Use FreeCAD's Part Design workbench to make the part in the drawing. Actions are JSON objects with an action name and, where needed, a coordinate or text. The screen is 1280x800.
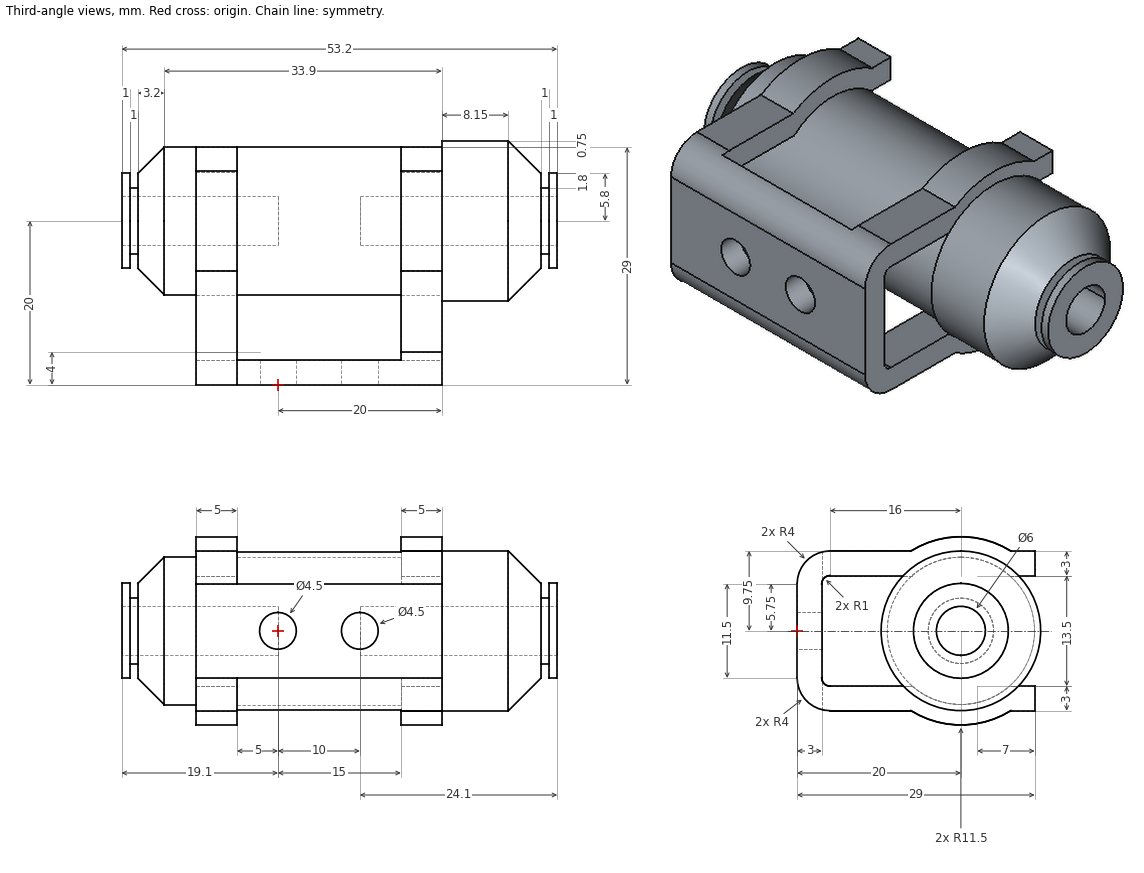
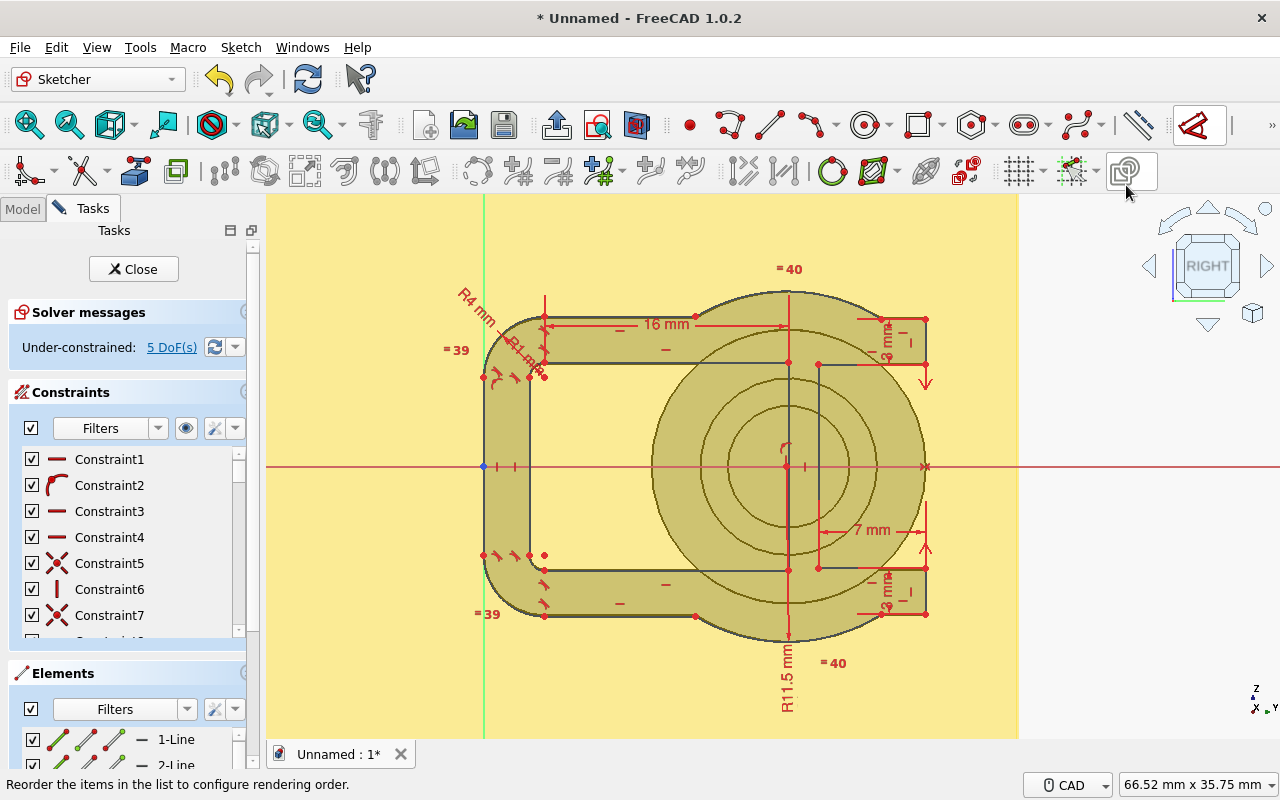
{"action": "left_click", "coordinate": [926, 614]}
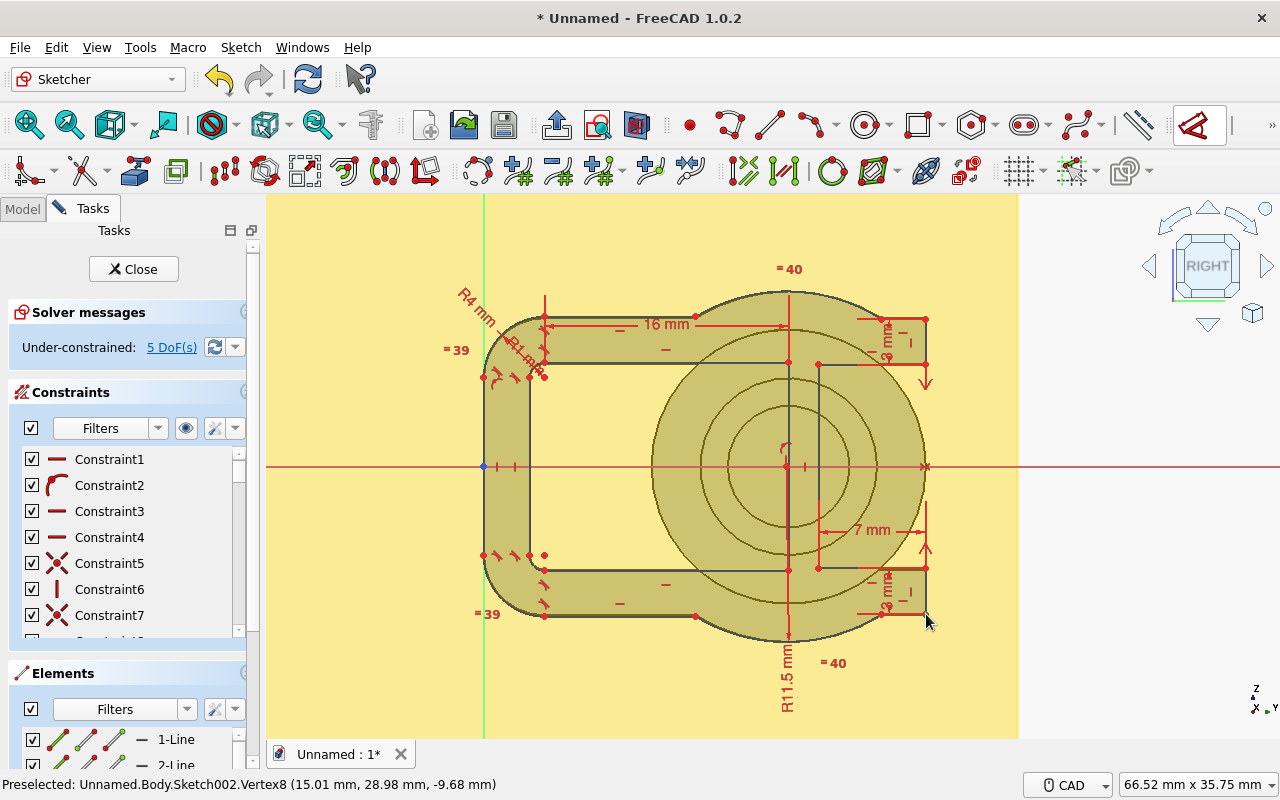
{"action": "left_click", "coordinate": [1220, 126]}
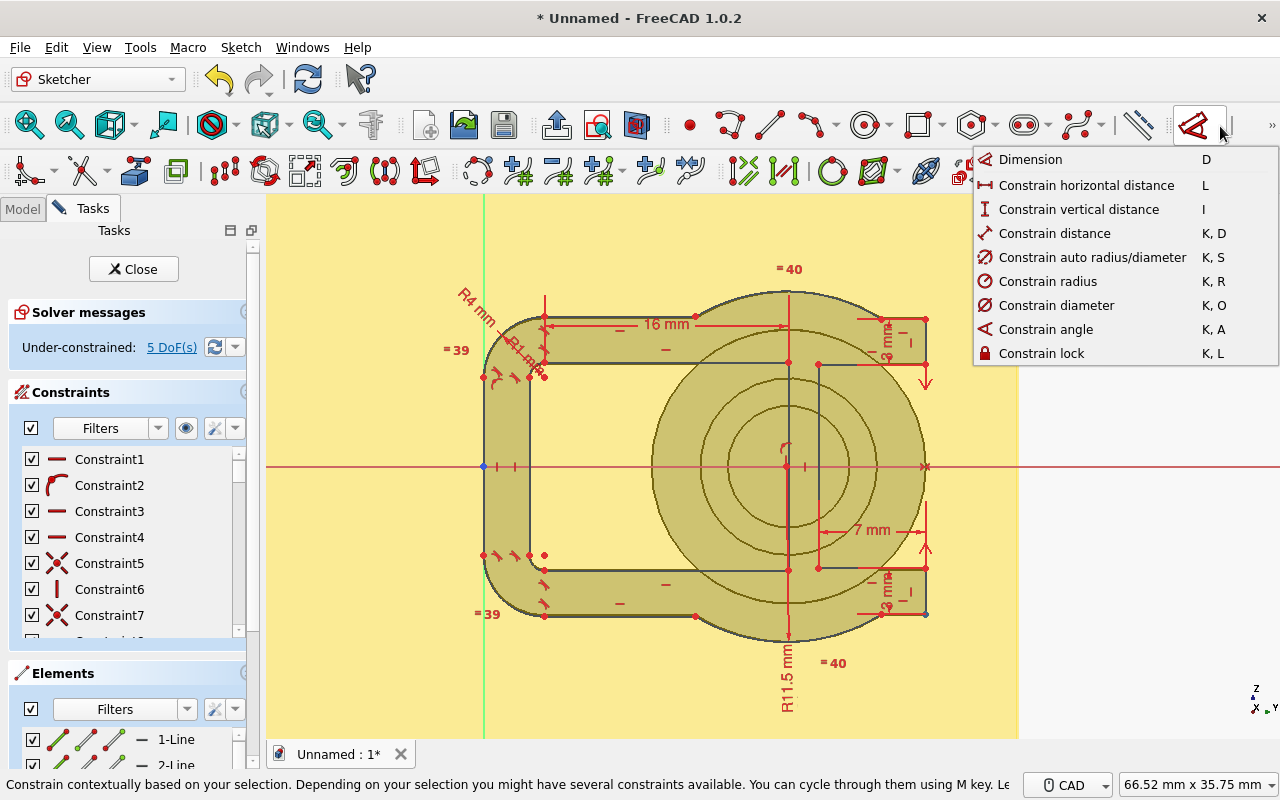
{"action": "left_click", "coordinate": [1126, 185]}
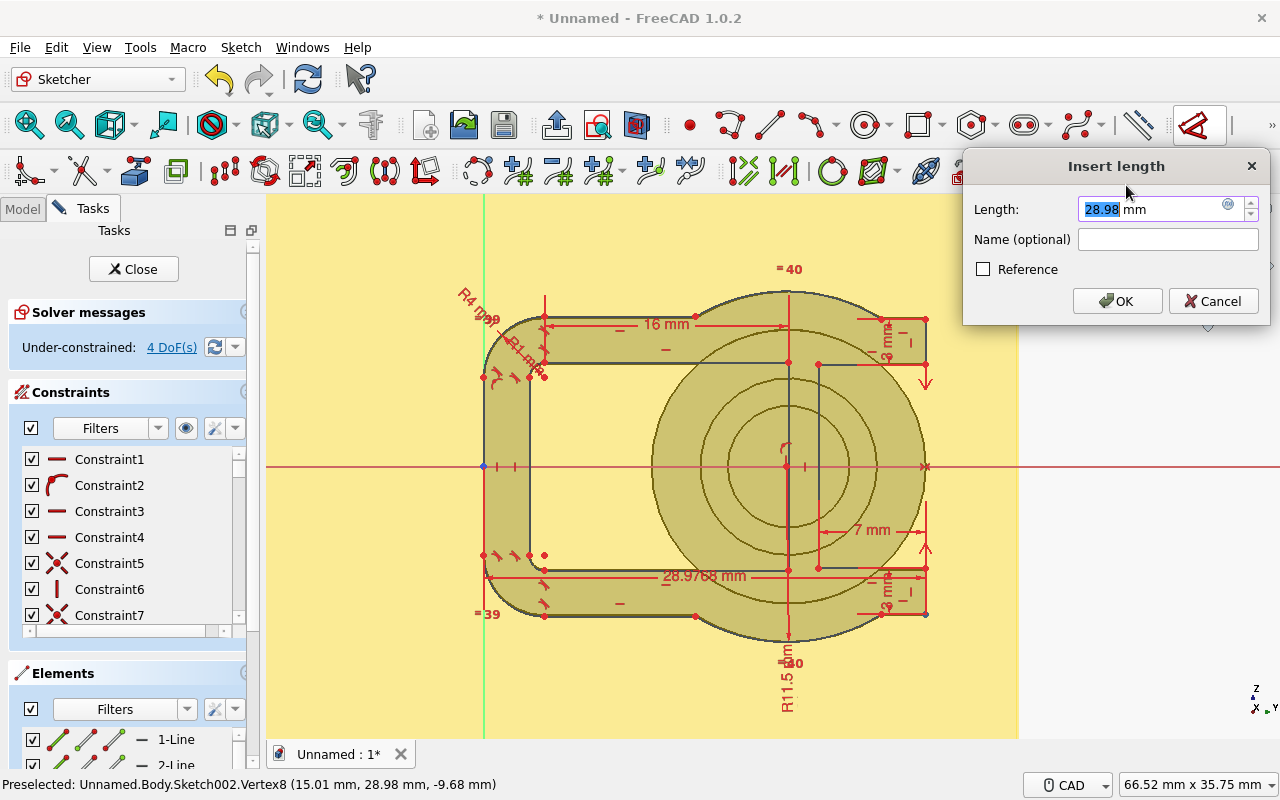
{"action": "type", "text": "29"}
{"action": "key", "text": "Return"}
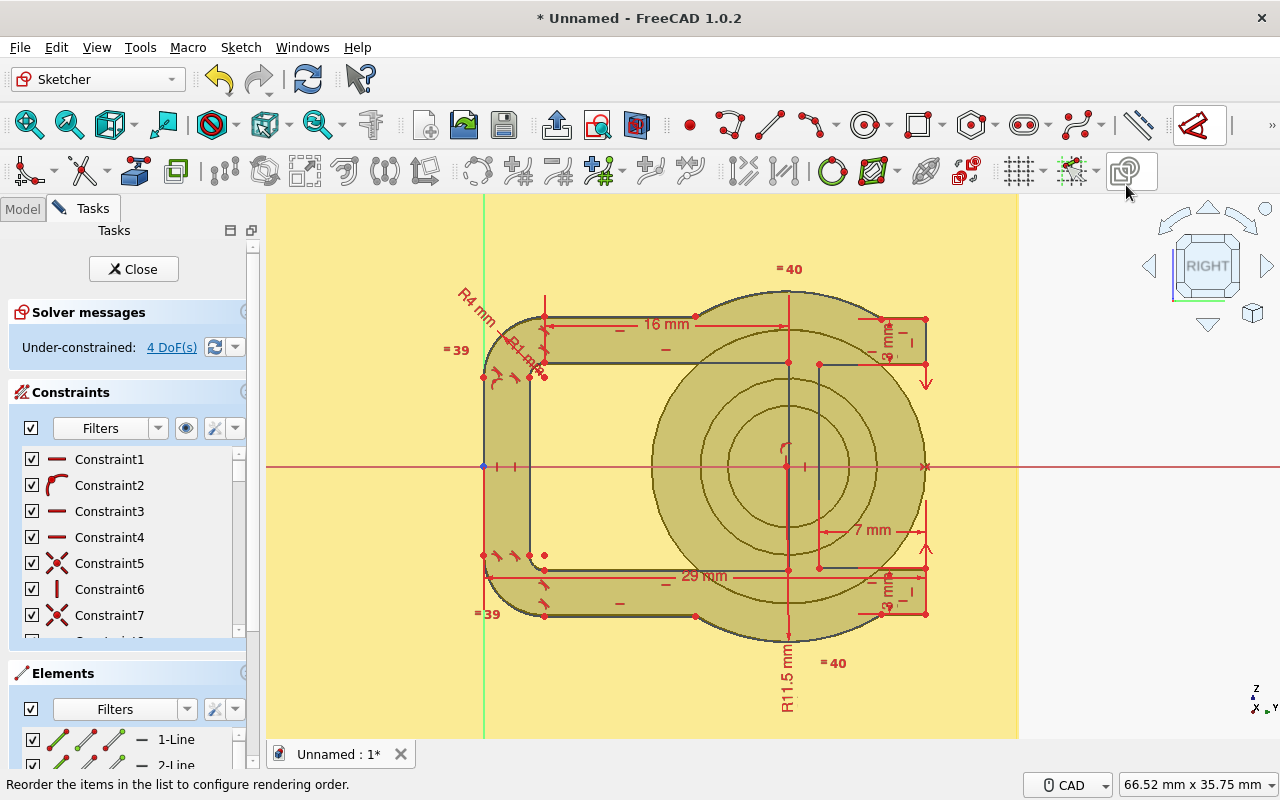
{"action": "left_click", "coordinate": [787, 467]}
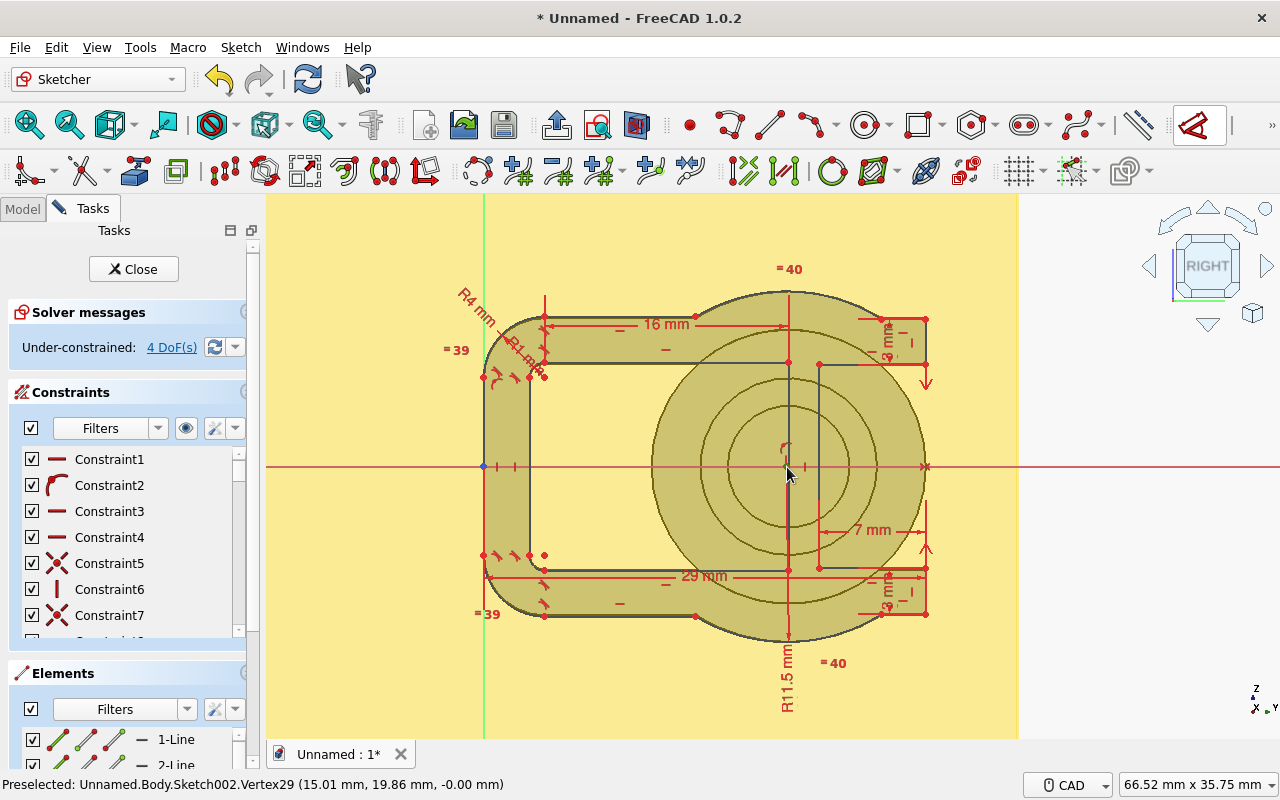
{"action": "key", "text": "l"}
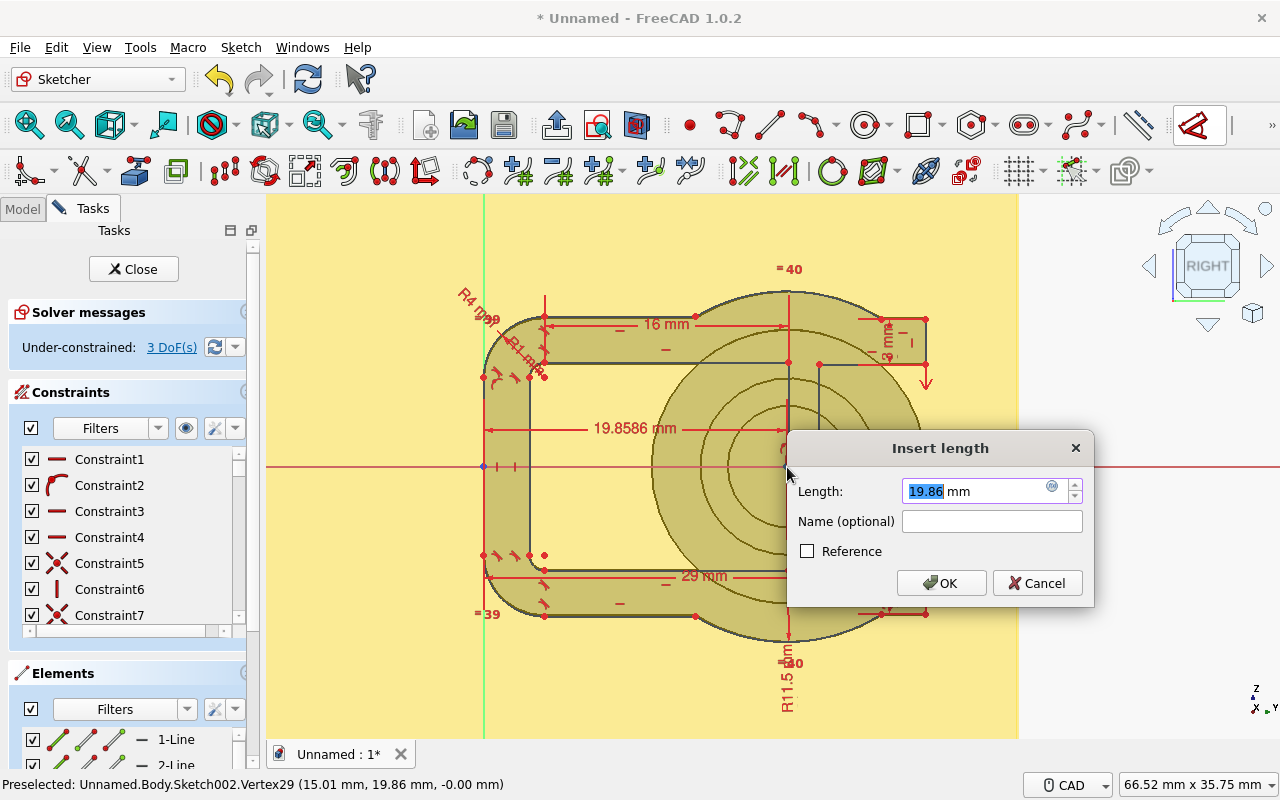
{"action": "type", "text": "20"}
{"action": "key", "text": "Return"}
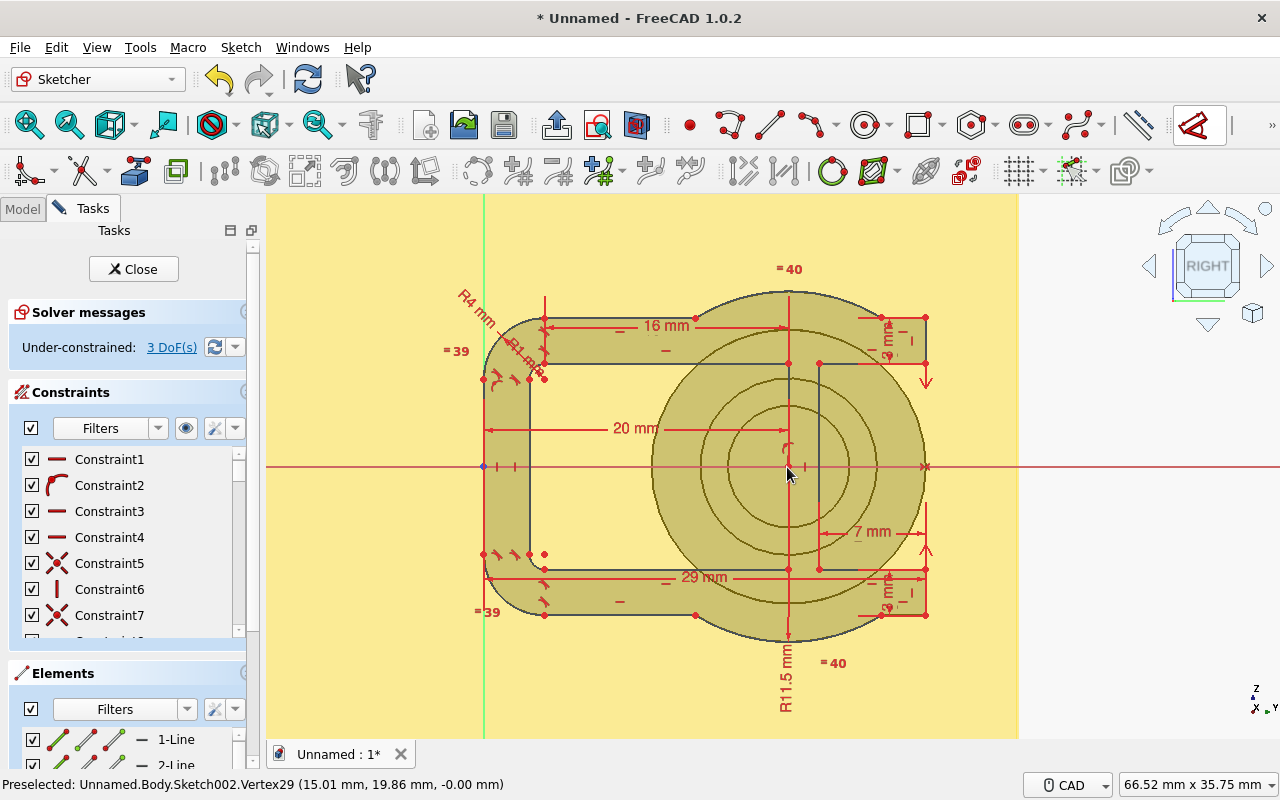
{"action": "left_click", "coordinate": [484, 432]}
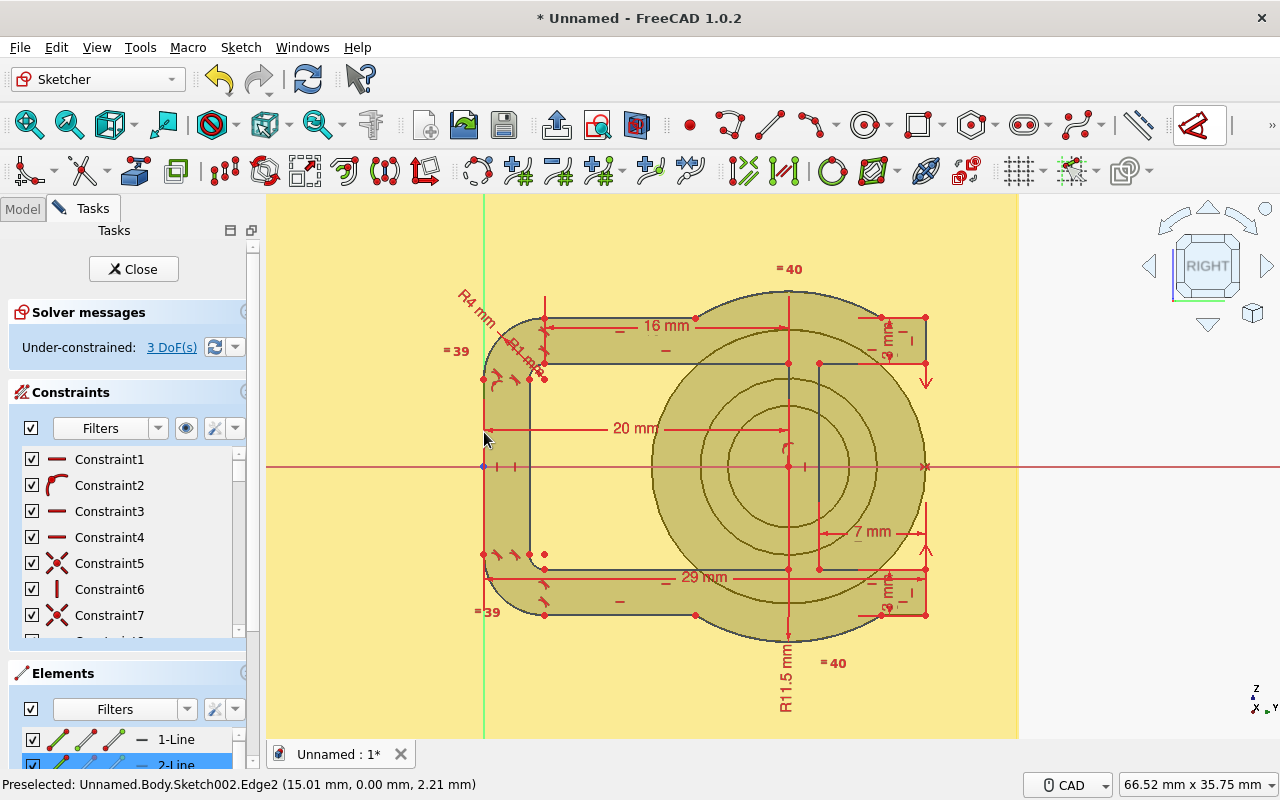
{"action": "left_click", "coordinate": [1220, 126]}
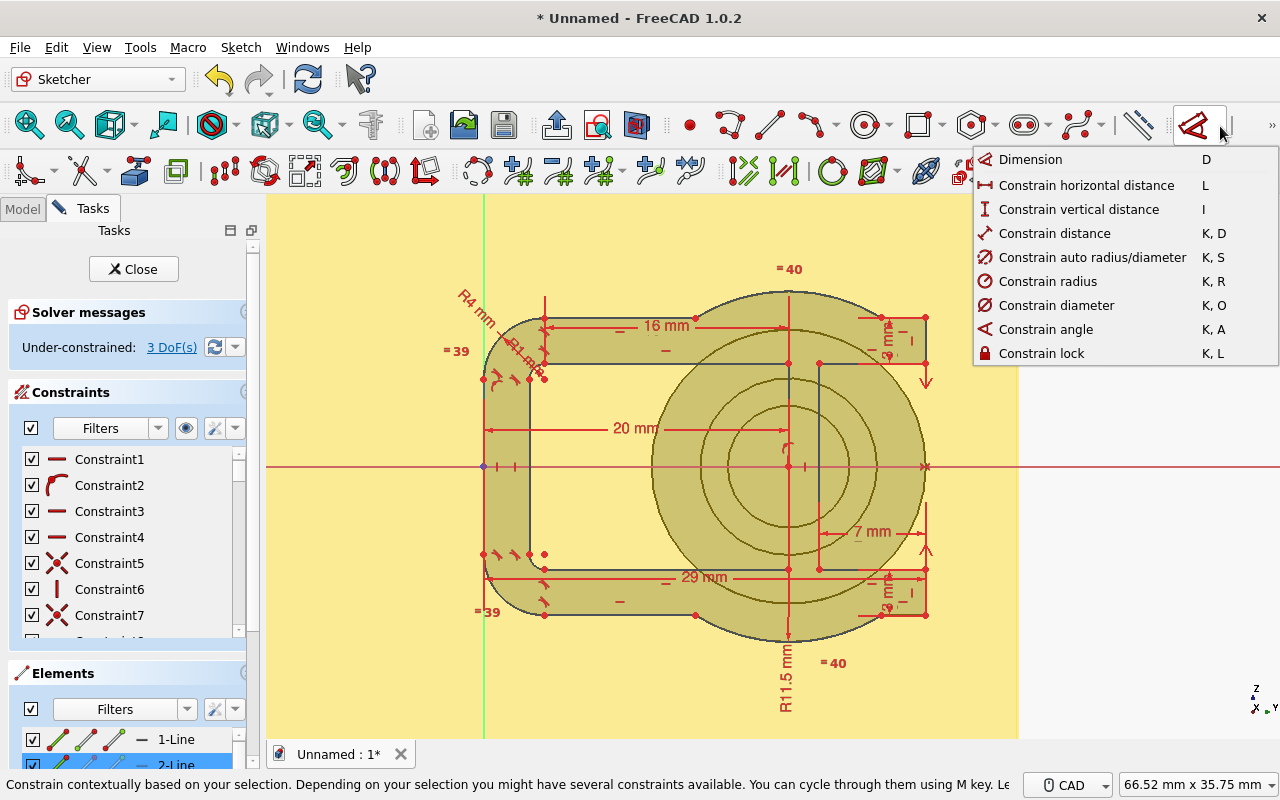
{"action": "left_click", "coordinate": [1126, 209]}